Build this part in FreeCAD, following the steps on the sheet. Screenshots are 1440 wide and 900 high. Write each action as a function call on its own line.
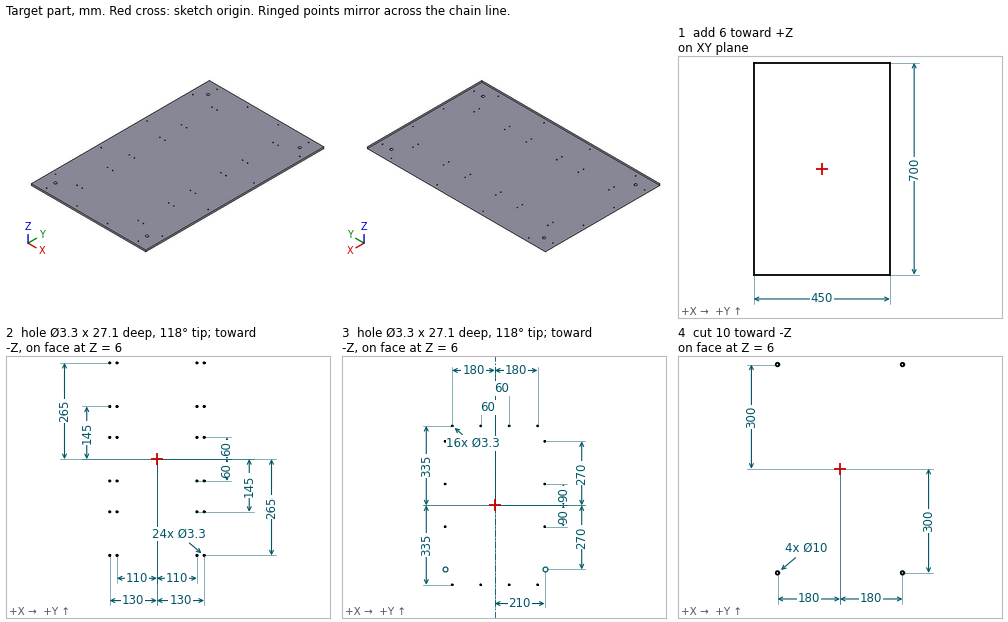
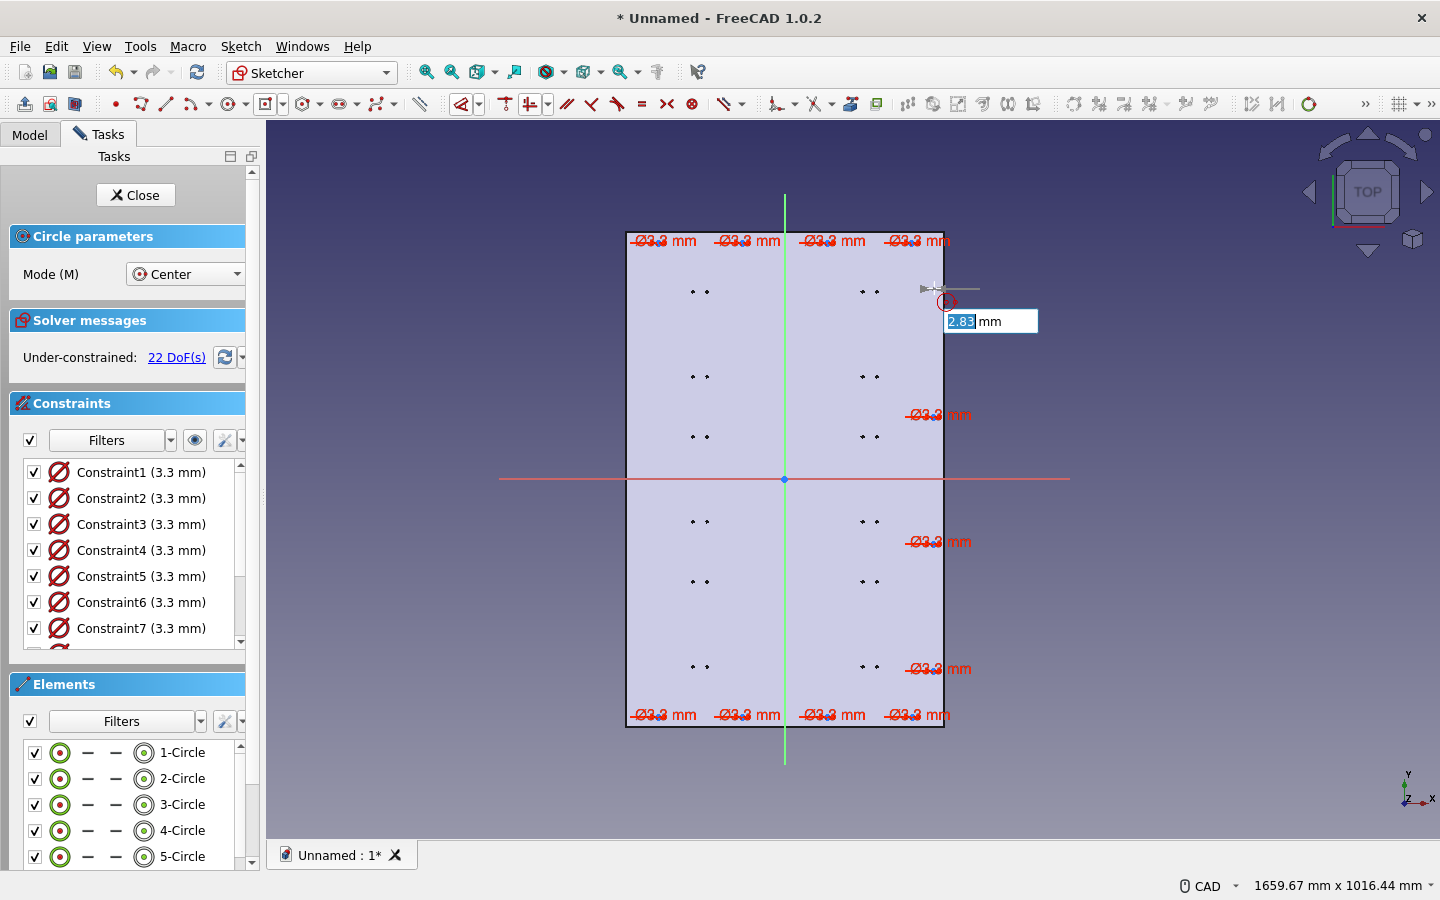
text(3.3)
key(Return)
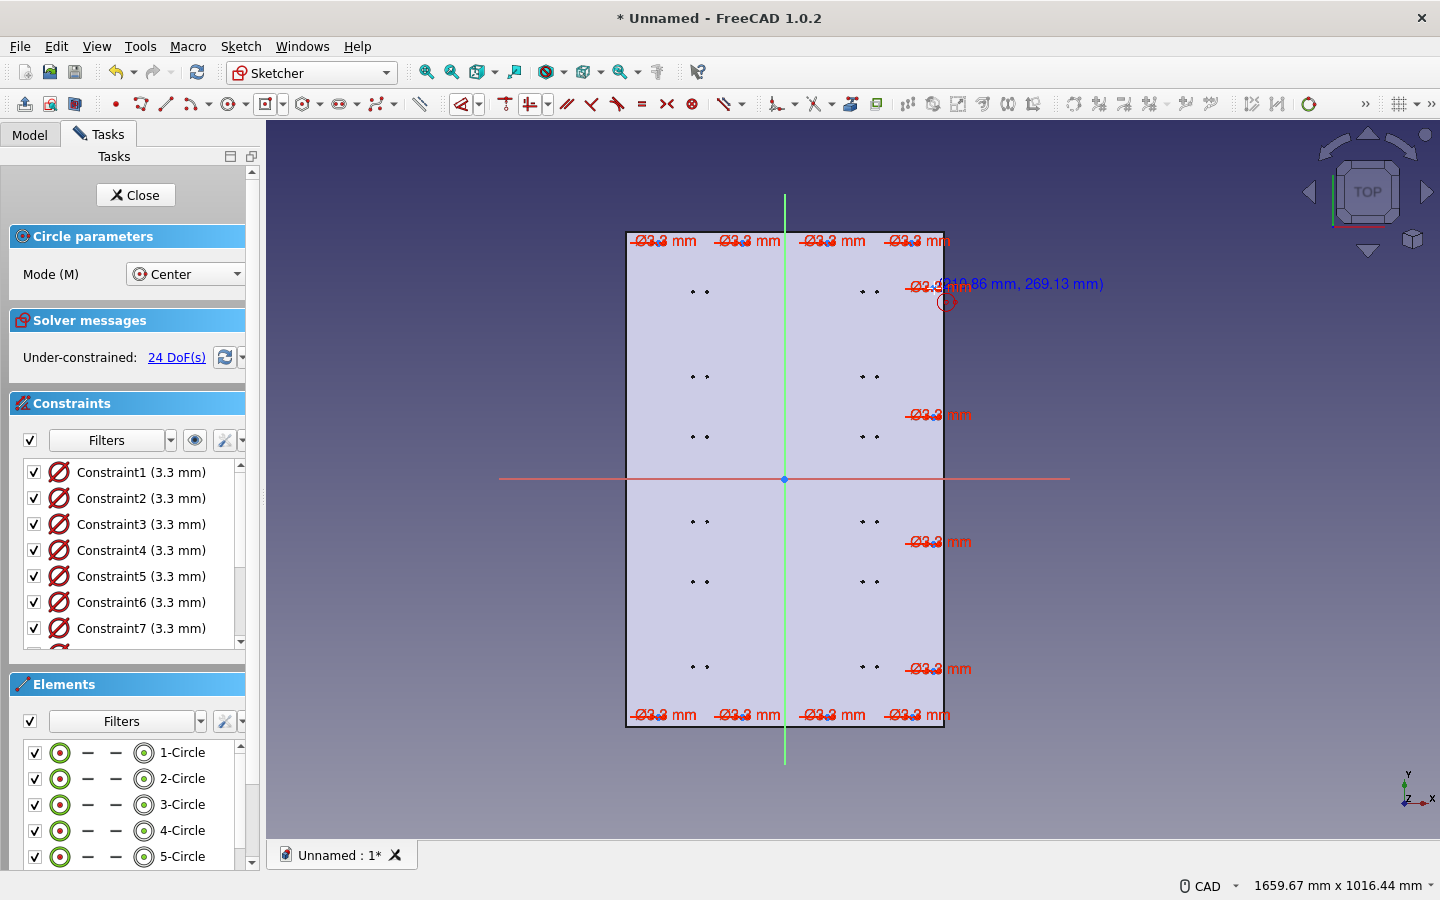
scroll(636, 288, up, 15)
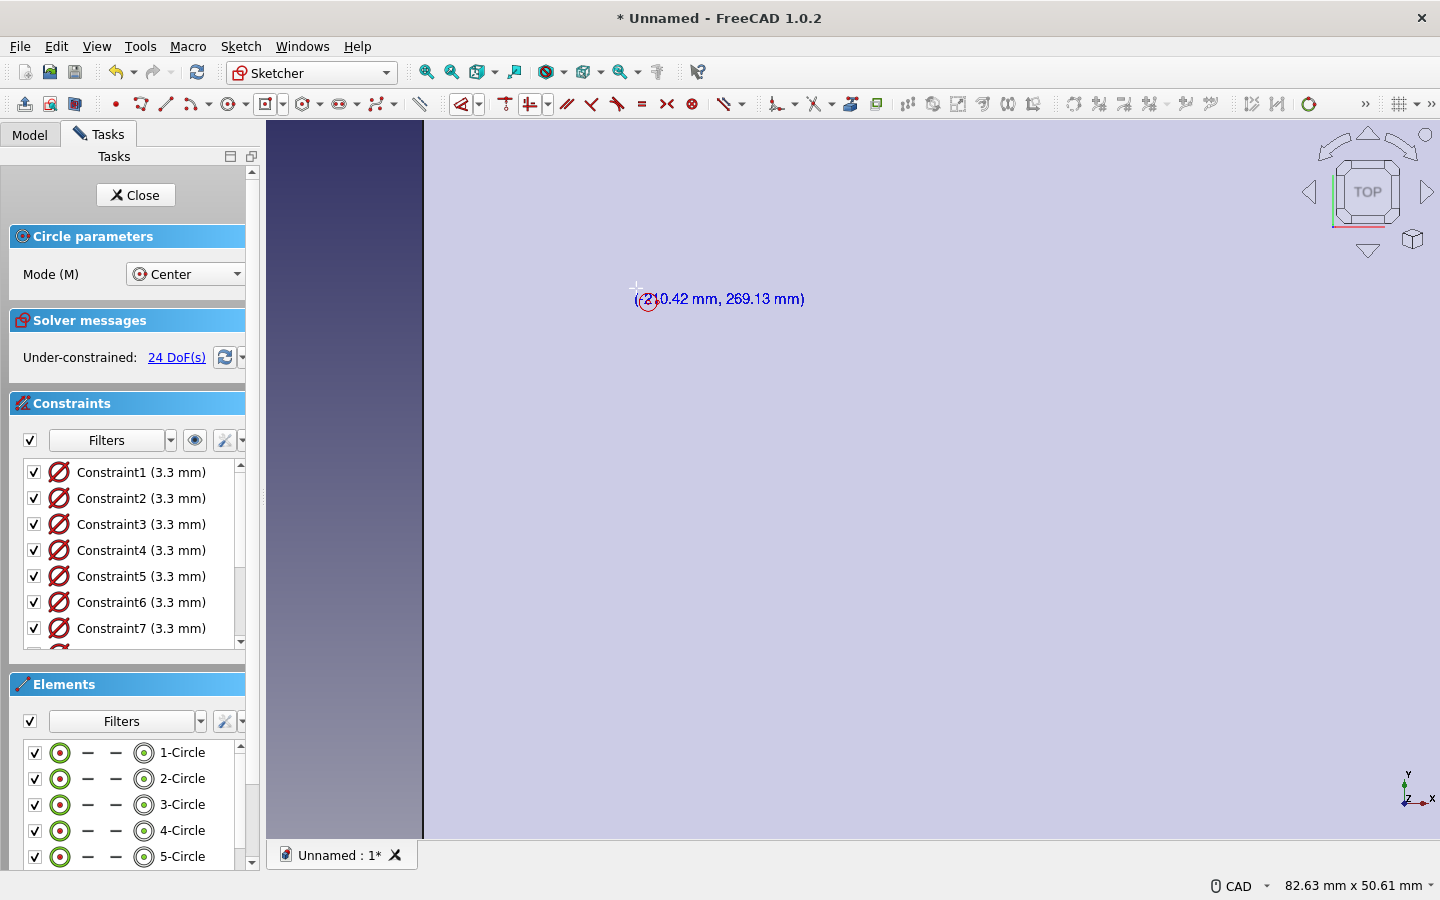
scroll(636, 288, down, 15)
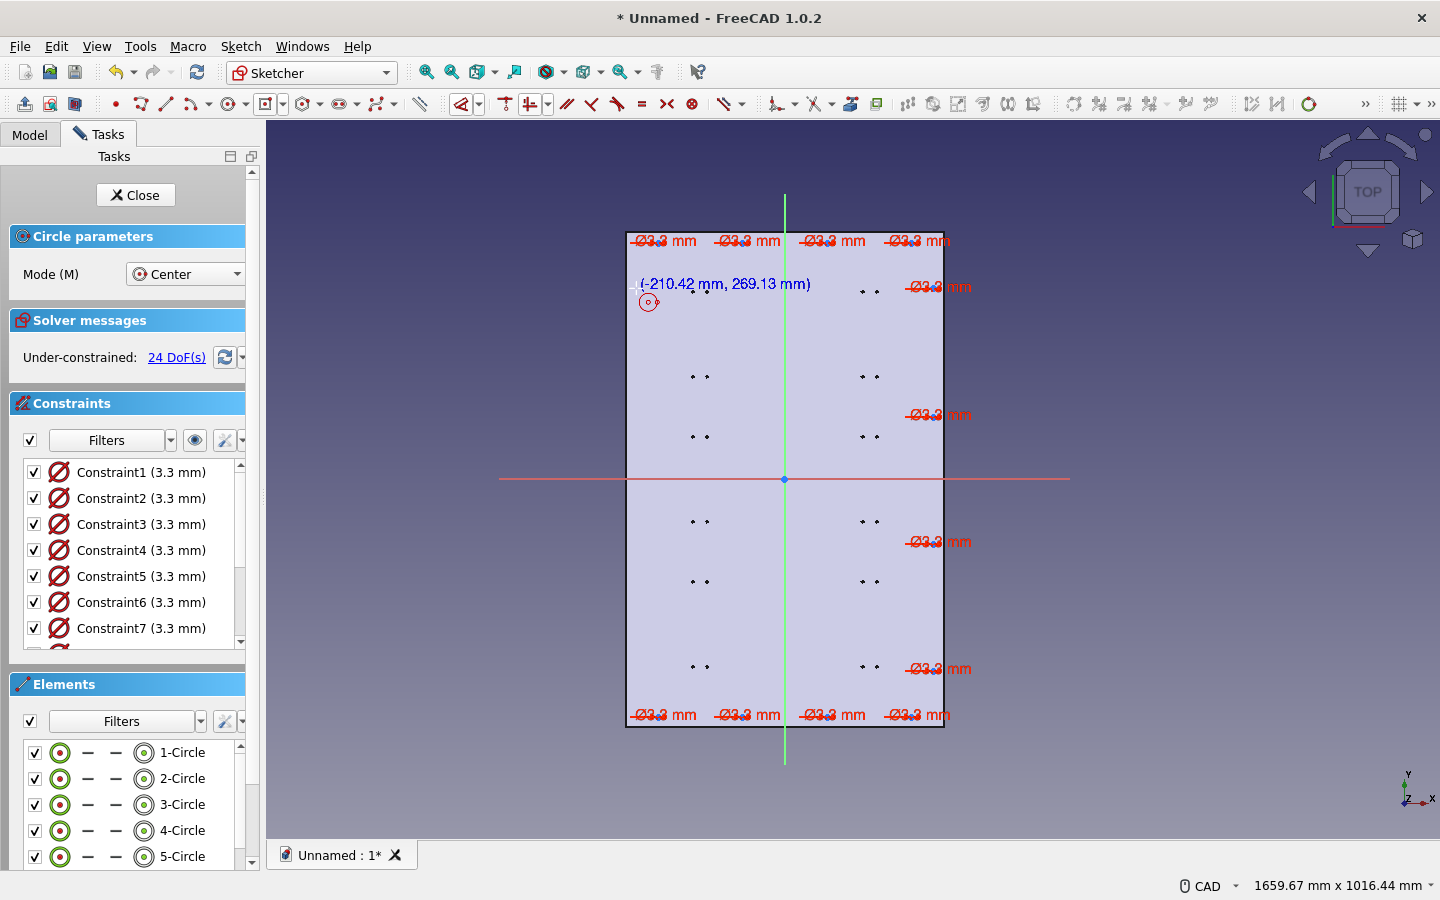
click(636, 288)
move(637, 288)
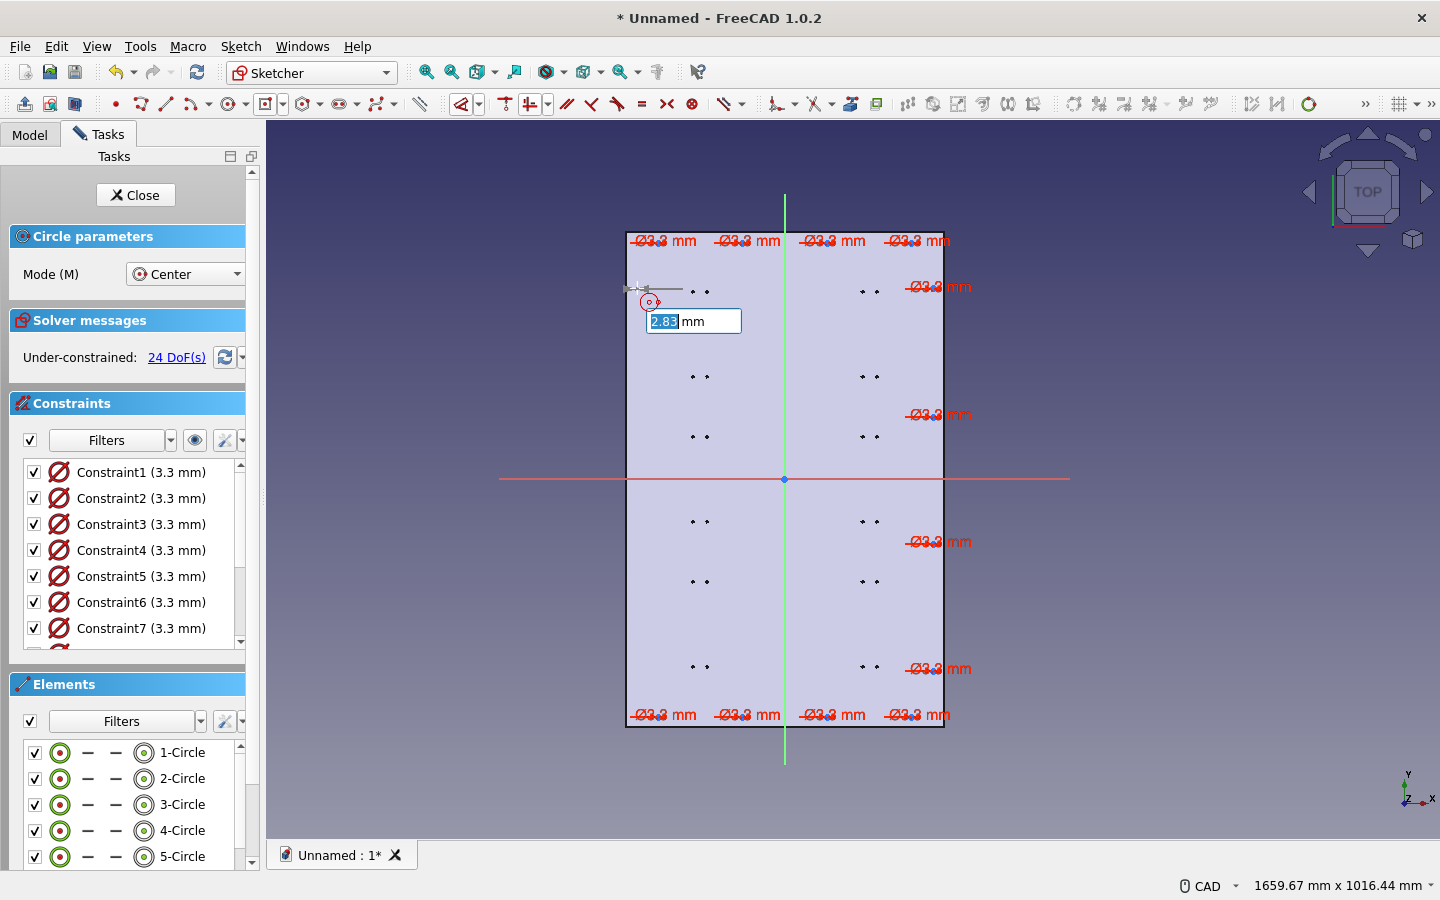
text(3.3)
key(Return)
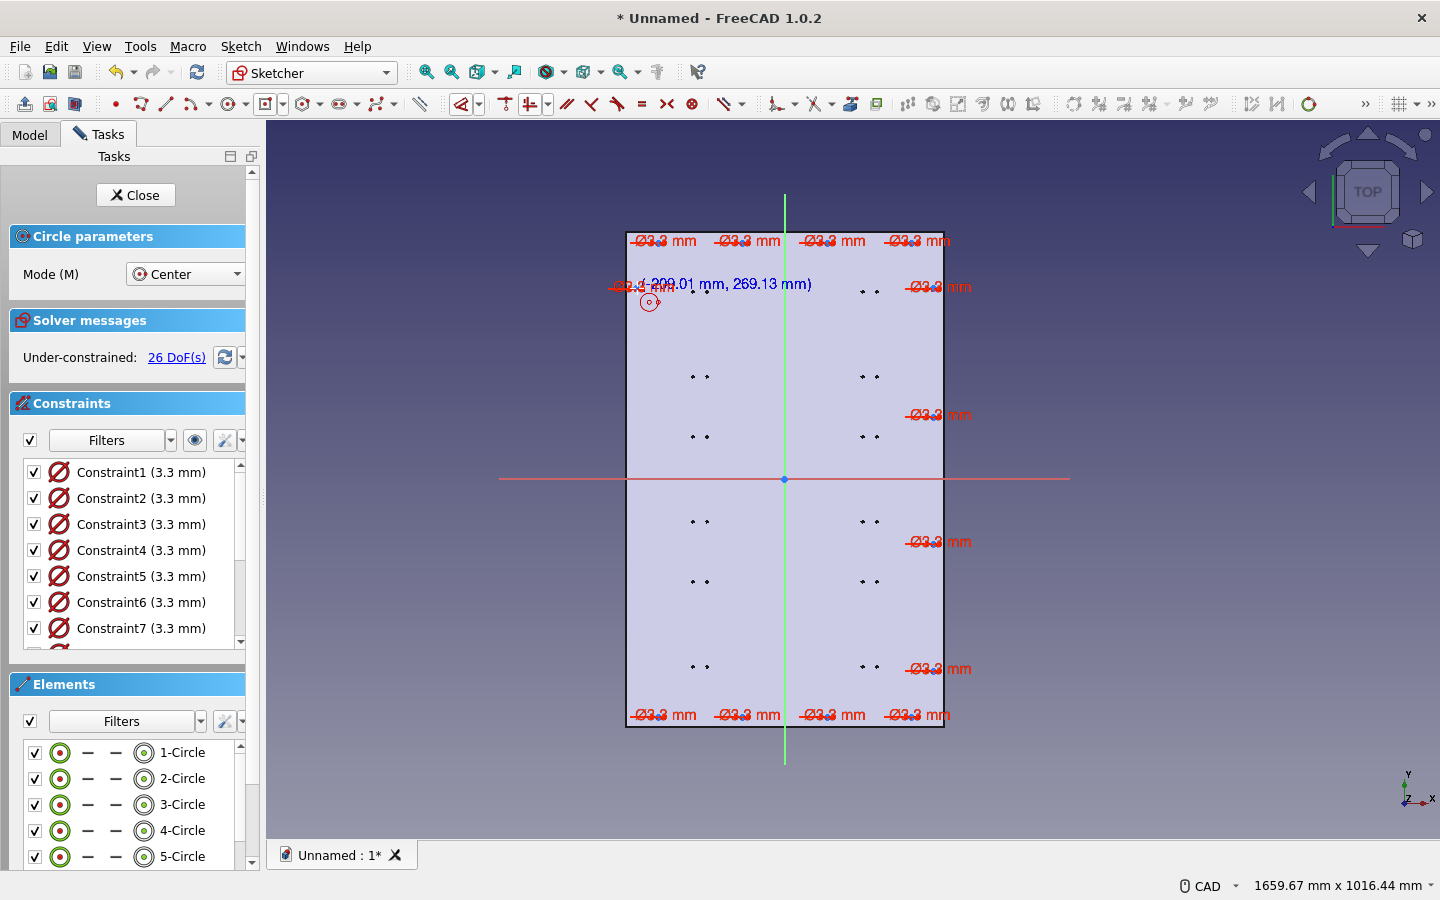
scroll(636, 416, up, 15)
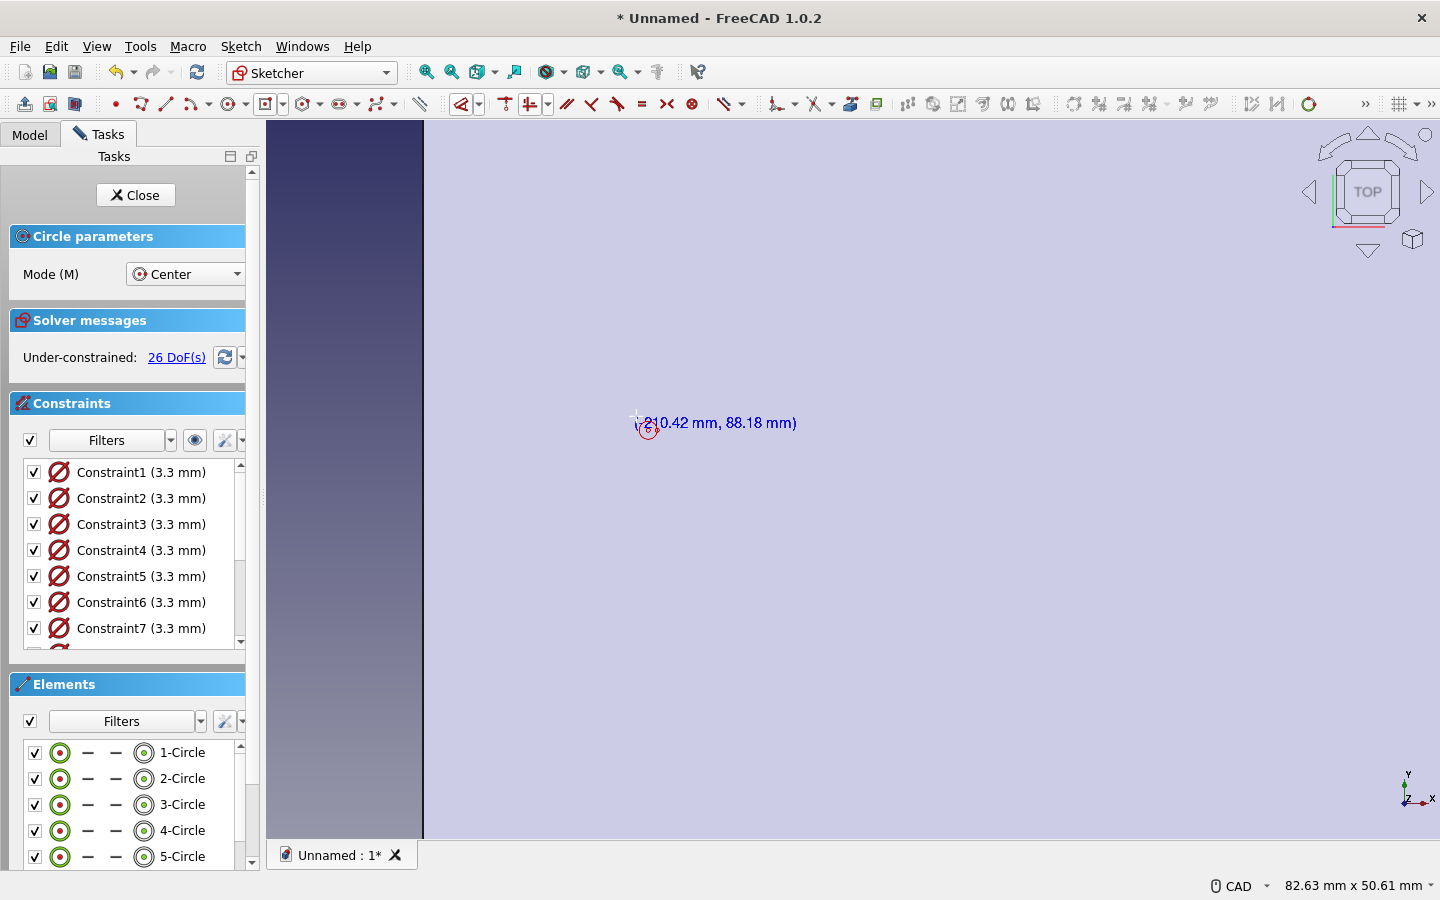
scroll(636, 417, down, 15)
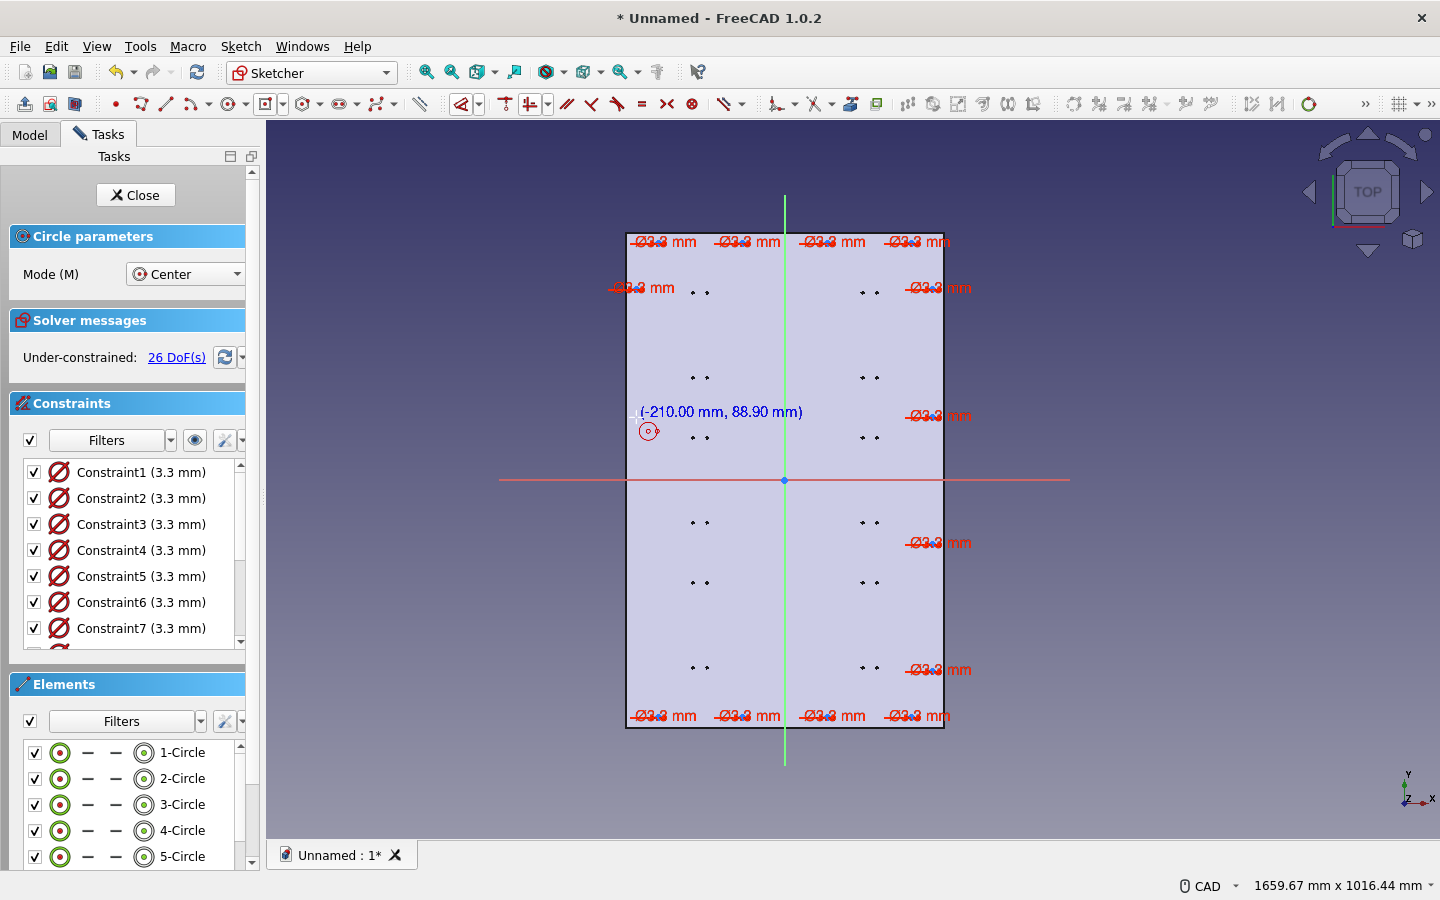
click(636, 417)
move(637, 416)